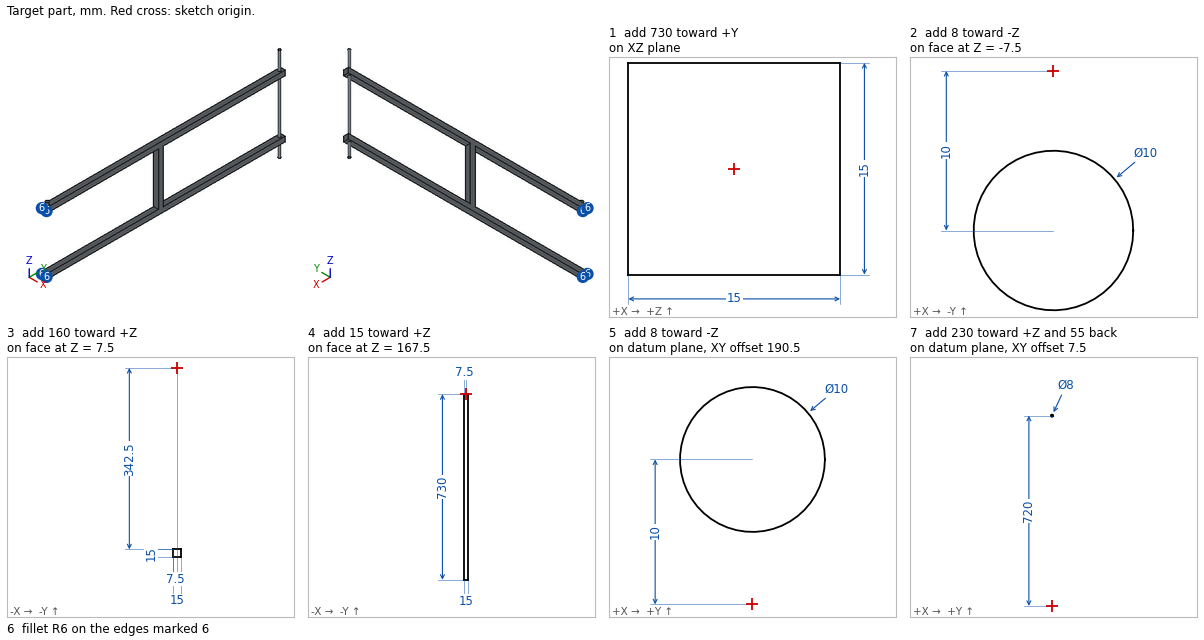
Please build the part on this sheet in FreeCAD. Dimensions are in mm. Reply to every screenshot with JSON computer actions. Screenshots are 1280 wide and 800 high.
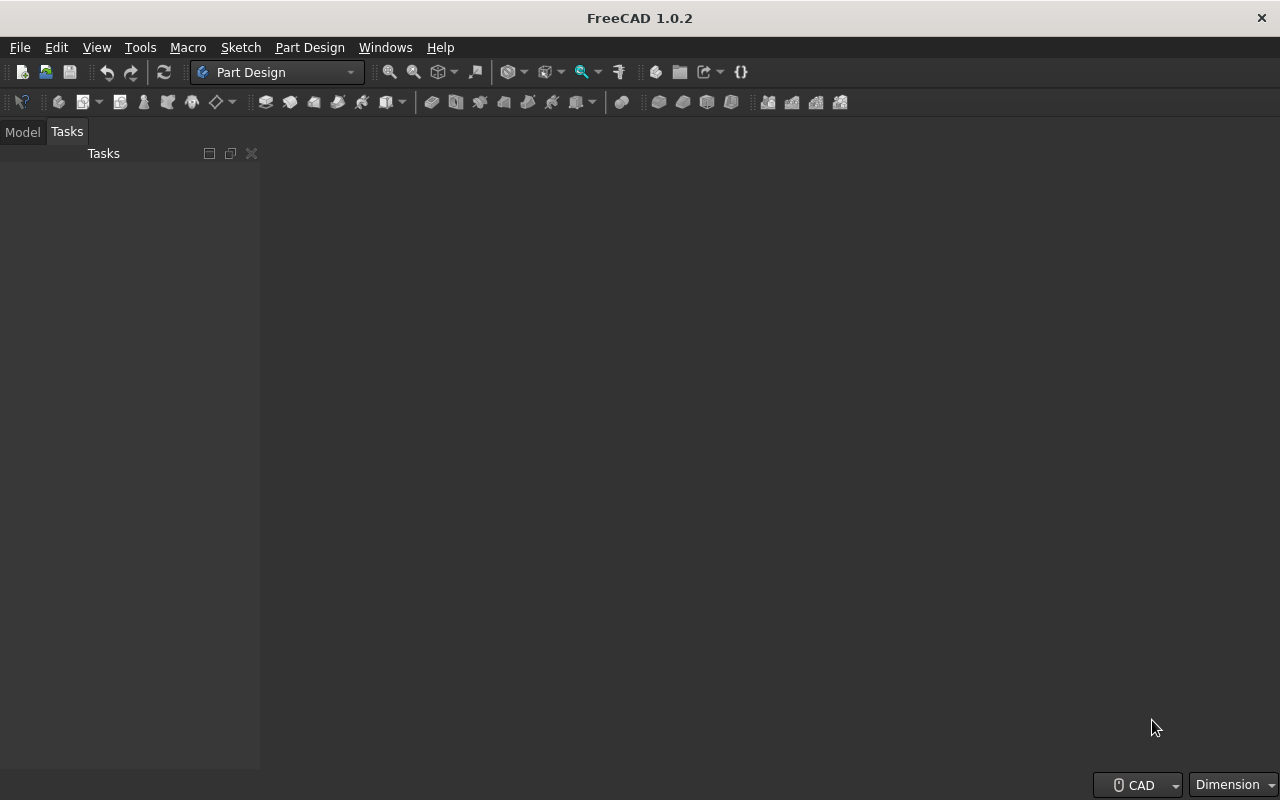
{"action": "left_click", "coordinate": [22, 72]}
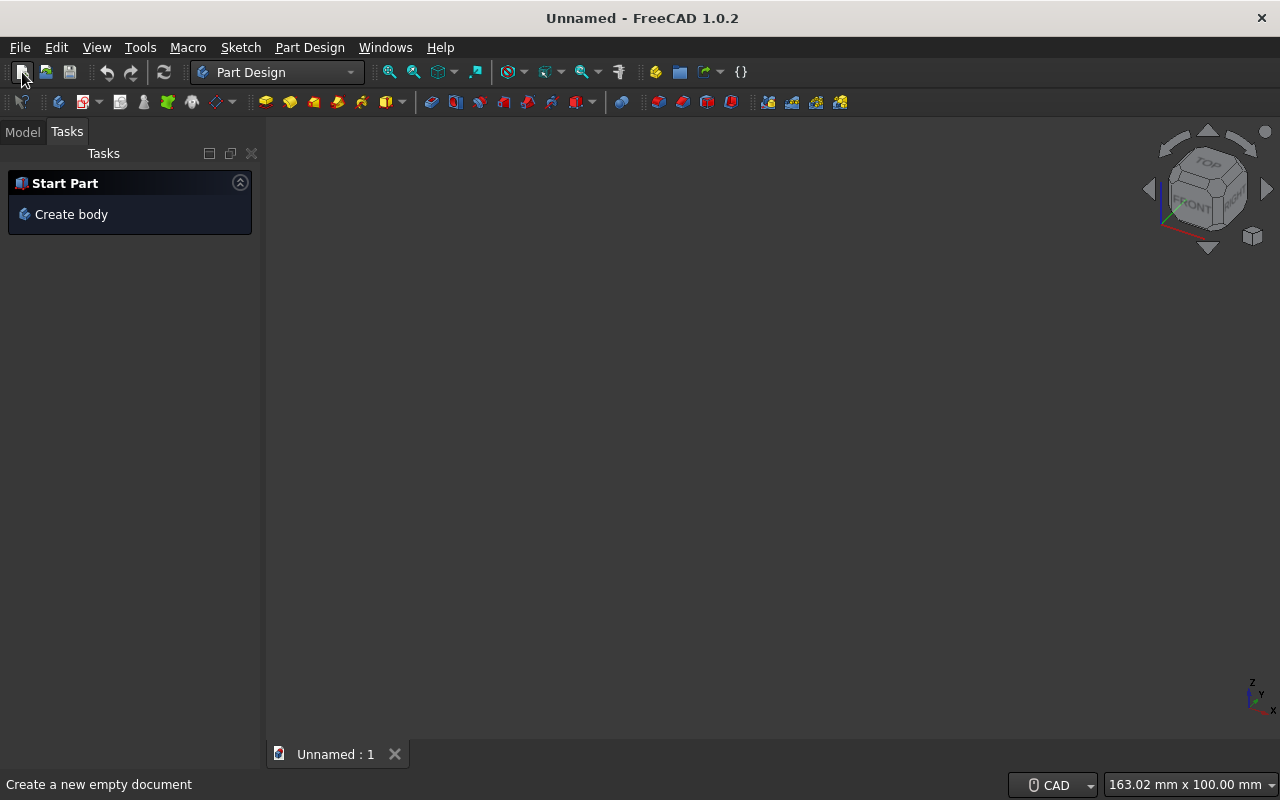
{"action": "left_click", "coordinate": [84, 102]}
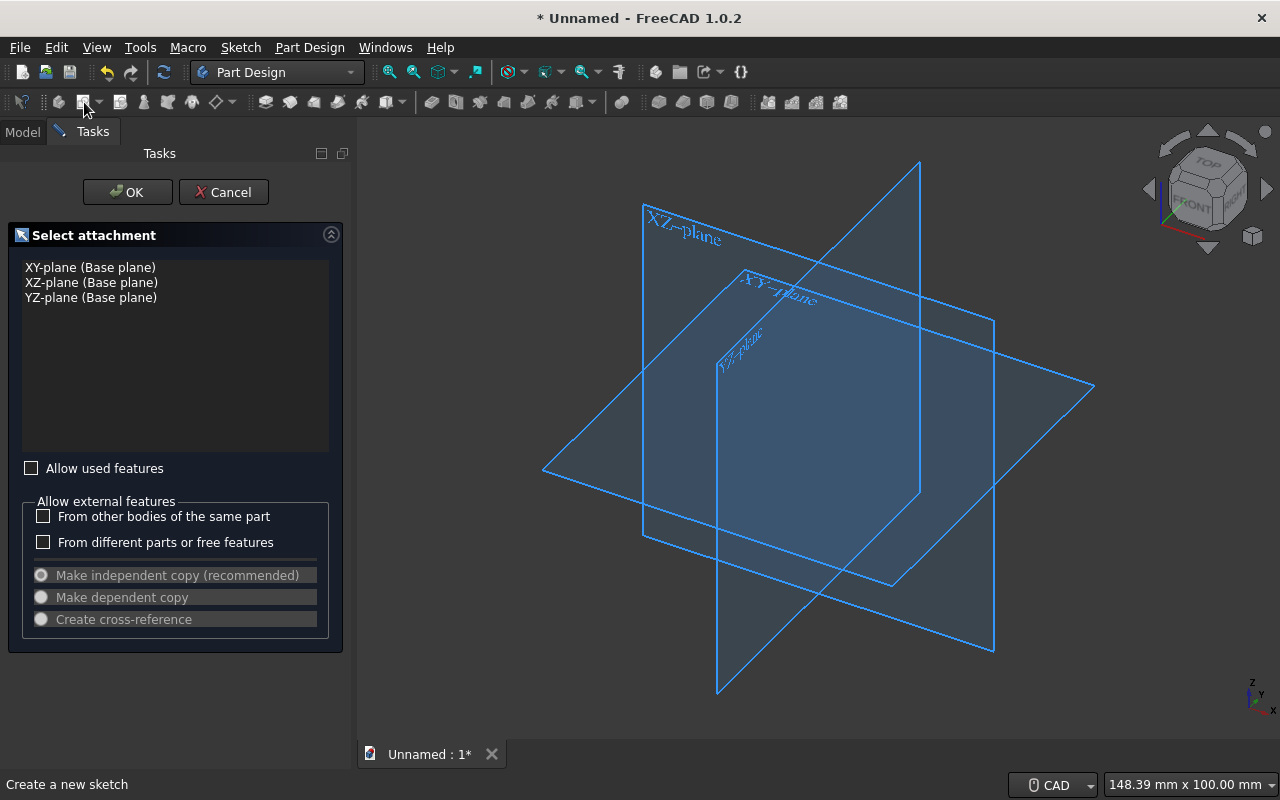
{"action": "left_click", "coordinate": [82, 282]}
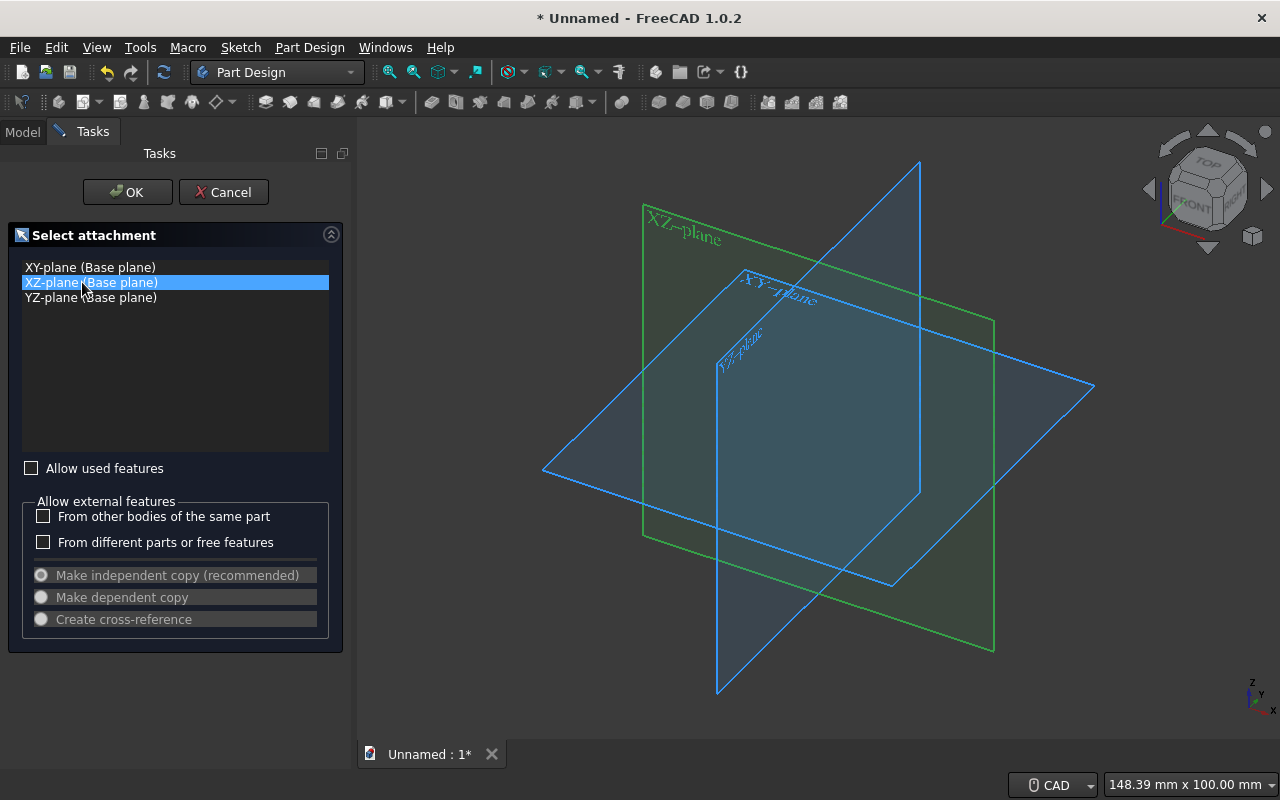
{"action": "left_click", "coordinate": [128, 192]}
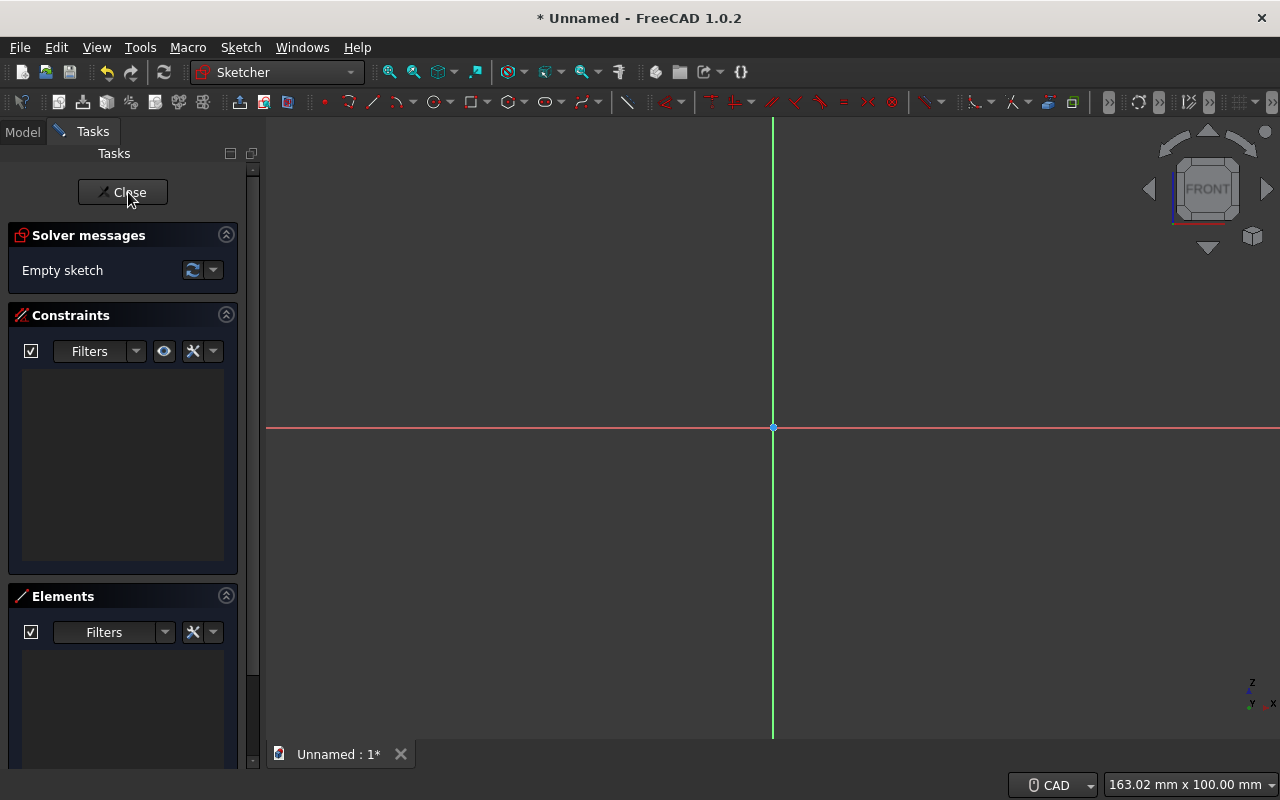
{"action": "scroll", "coordinate": [795, 428], "scroll_direction": "up", "scroll_amount": 7}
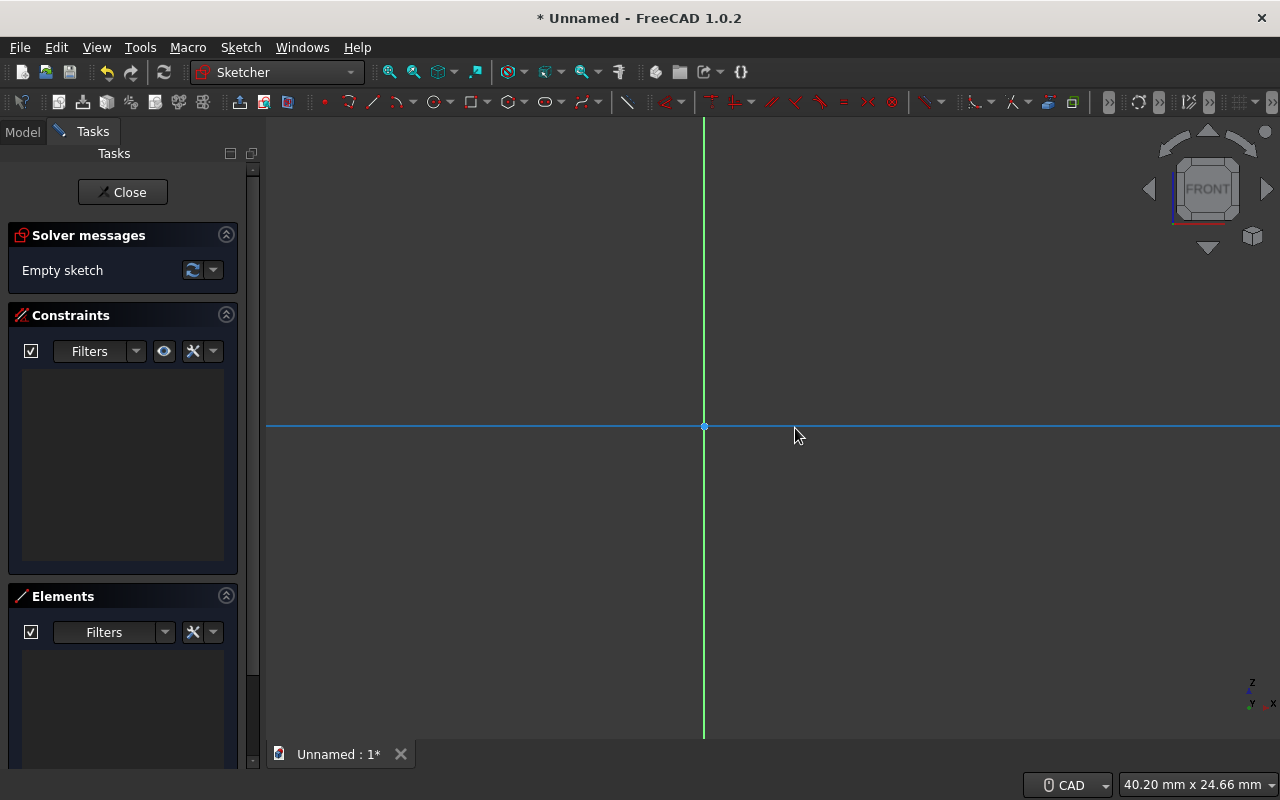
{"action": "left_click", "coordinate": [490, 102]}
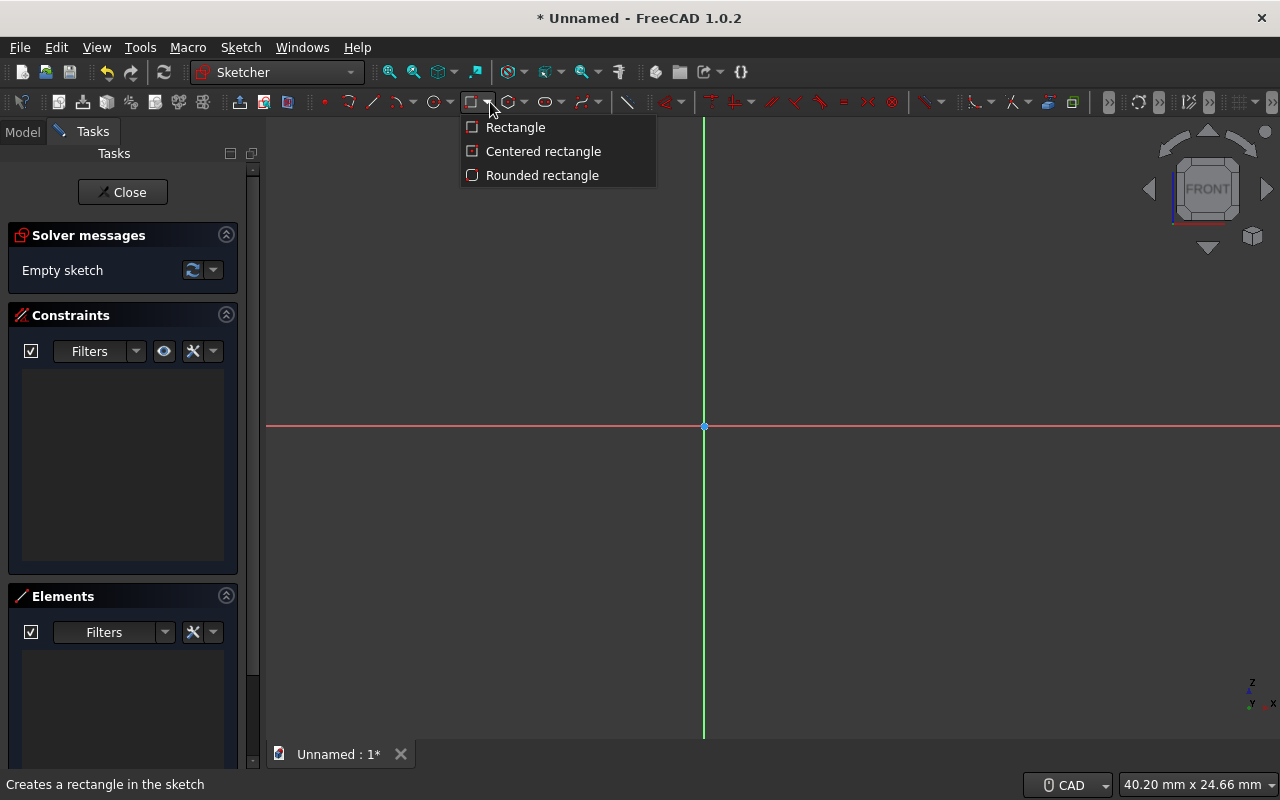
{"action": "left_click", "coordinate": [558, 151]}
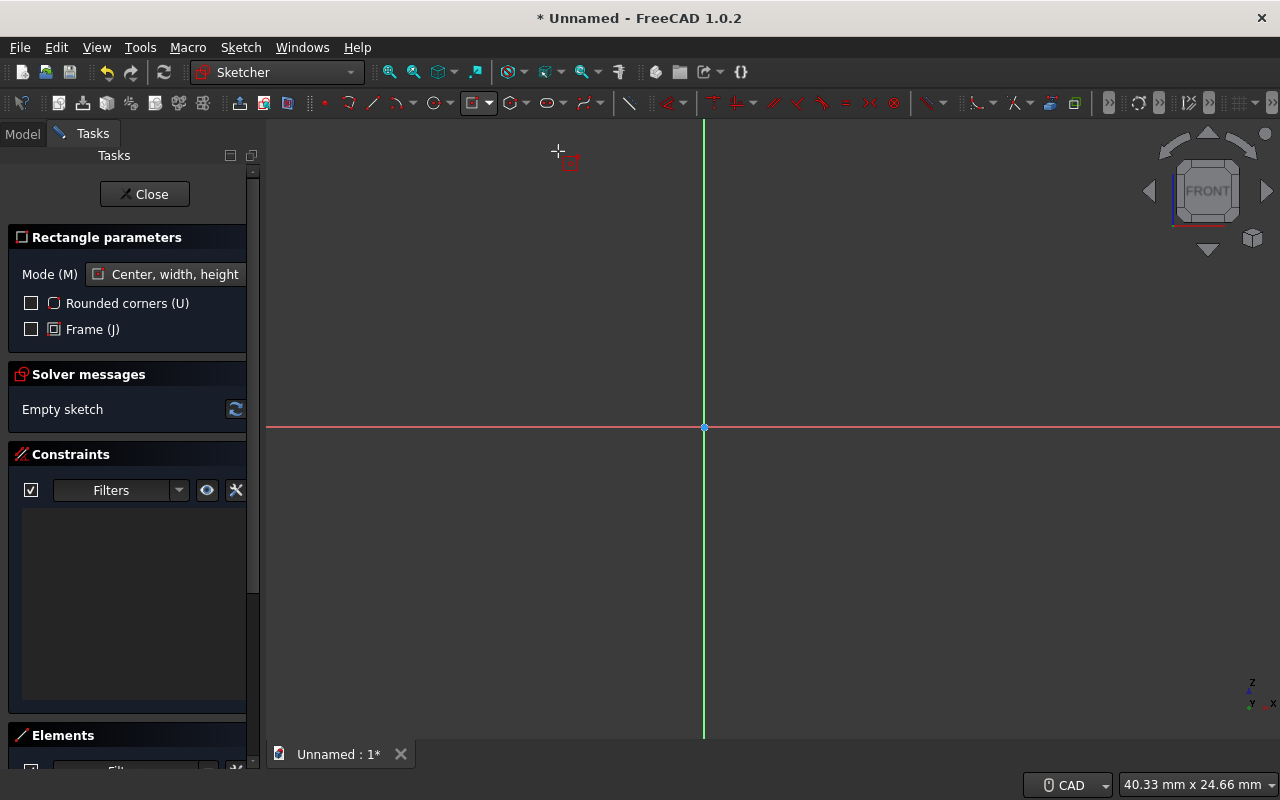
{"action": "left_click", "coordinate": [704, 427]}
{"action": "left_click", "coordinate": [893, 239]}
{"action": "key", "text": "Escape"}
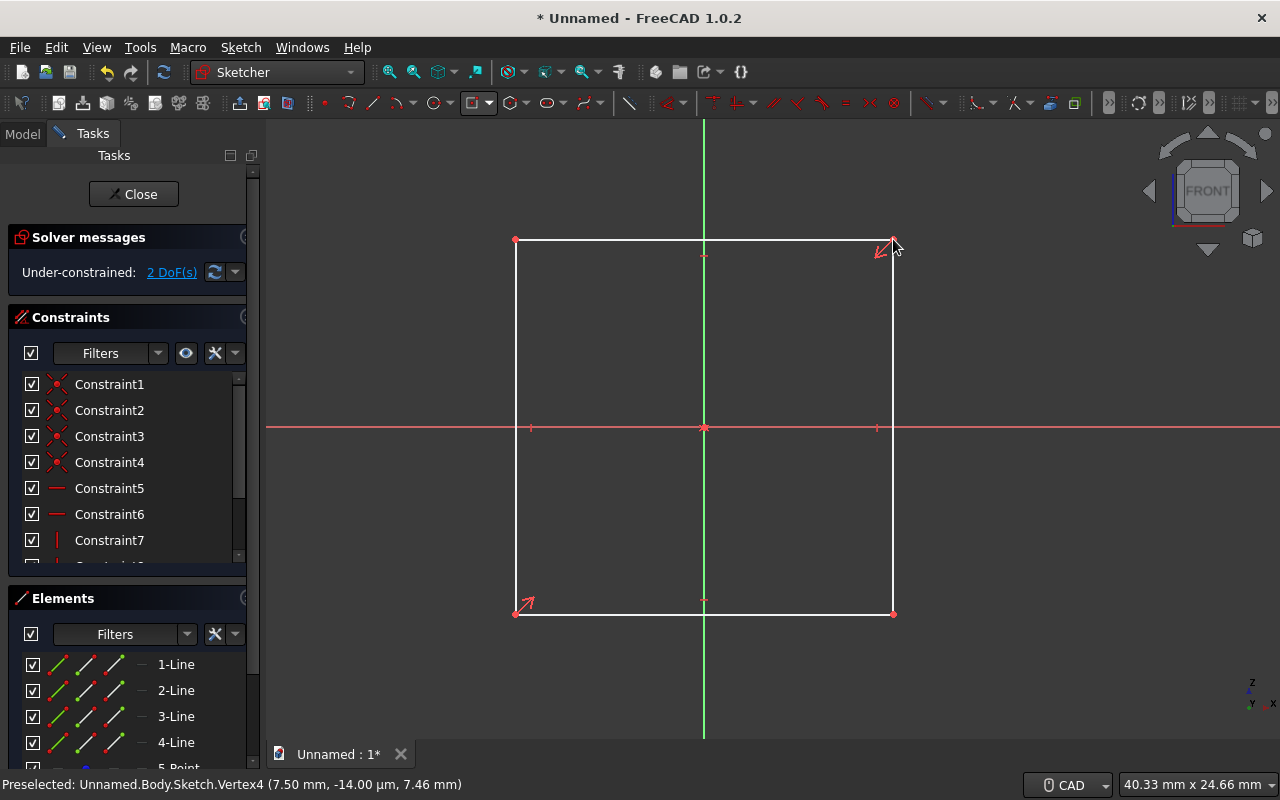
{"action": "left_click", "coordinate": [668, 104]}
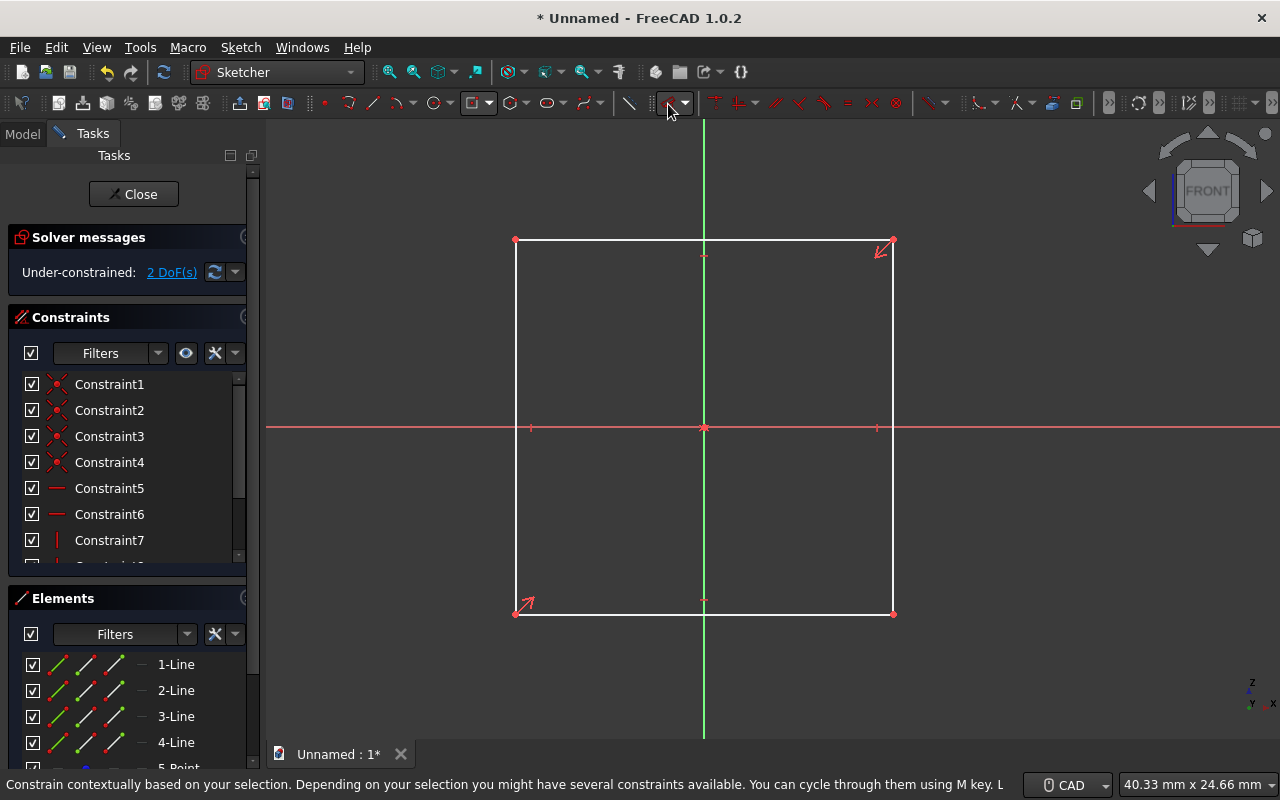
{"action": "left_click", "coordinate": [629, 615]}
{"action": "left_click", "coordinate": [618, 649]}